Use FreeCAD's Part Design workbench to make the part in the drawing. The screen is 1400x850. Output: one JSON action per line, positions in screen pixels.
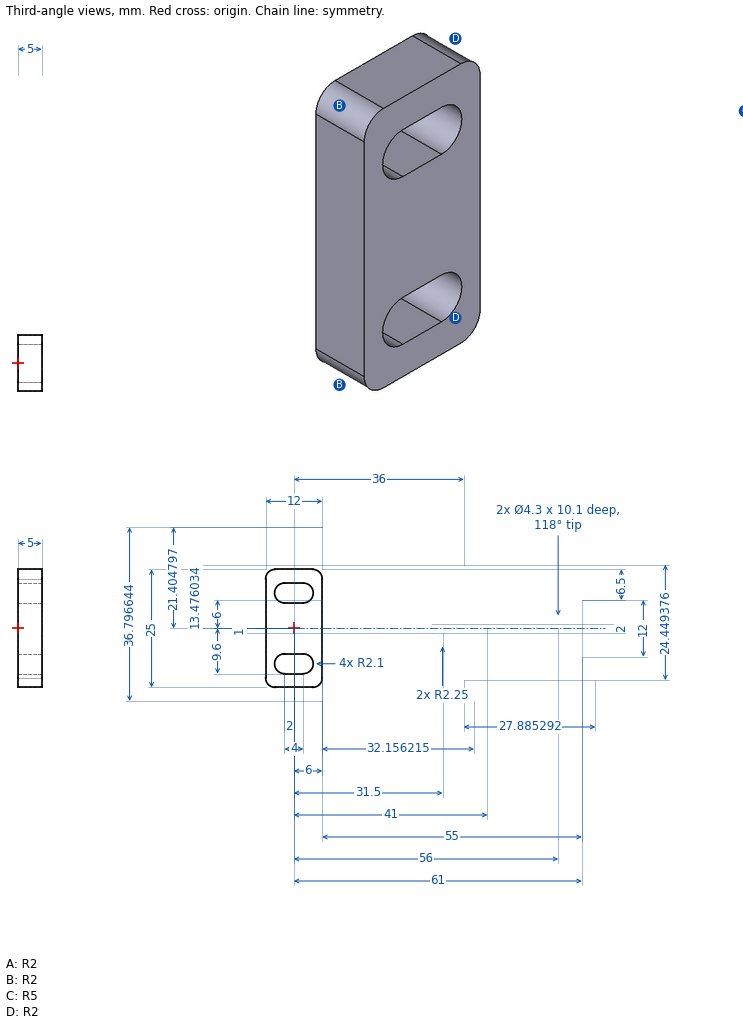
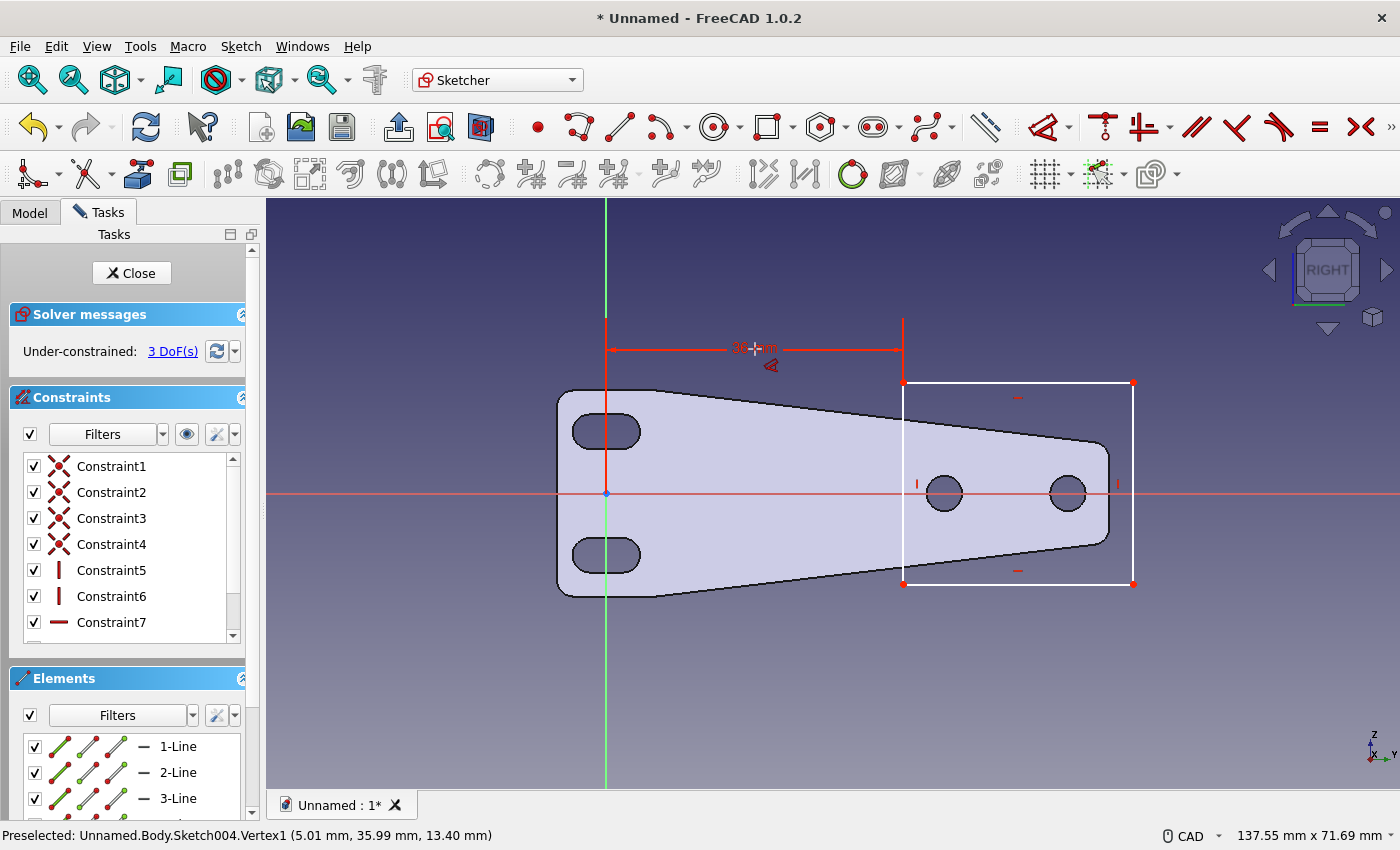
{"action": "left_click", "coordinate": [903, 444]}
{"action": "left_click", "coordinate": [937, 438]}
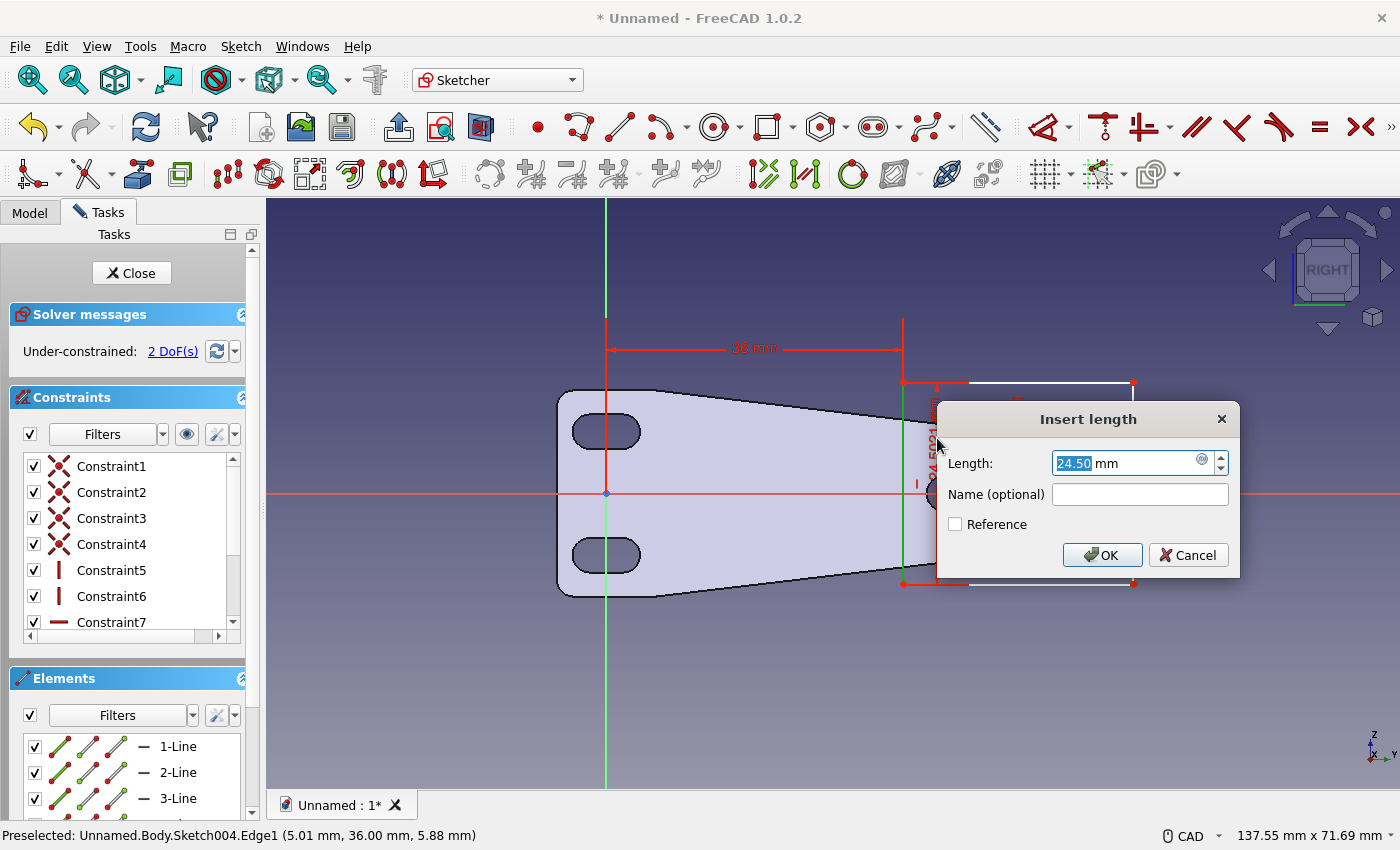
{"action": "type", "text": "24.449376"}
{"action": "key", "text": "Return"}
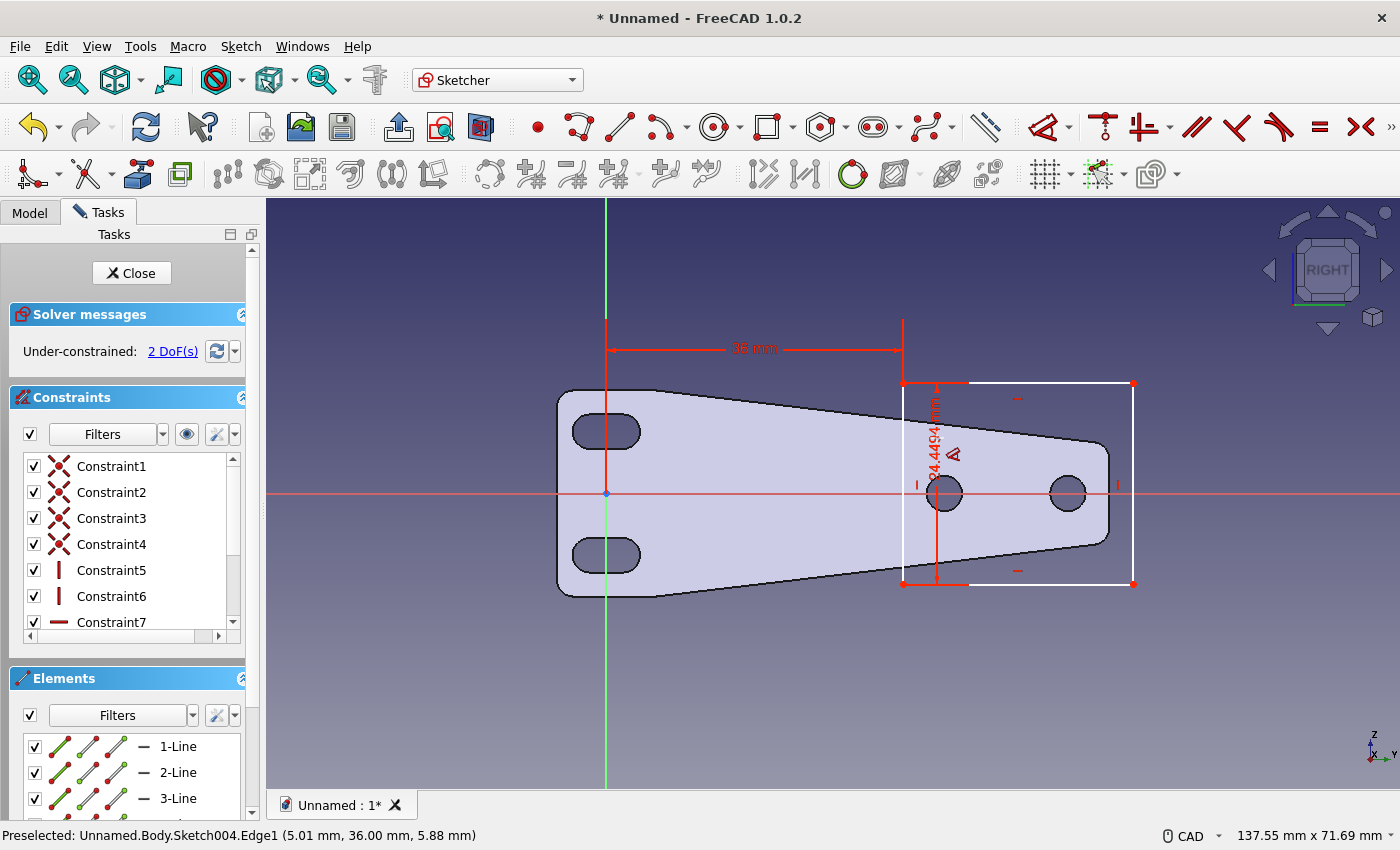
{"action": "left_click", "coordinate": [972, 585]}
{"action": "left_click", "coordinate": [1018, 619]}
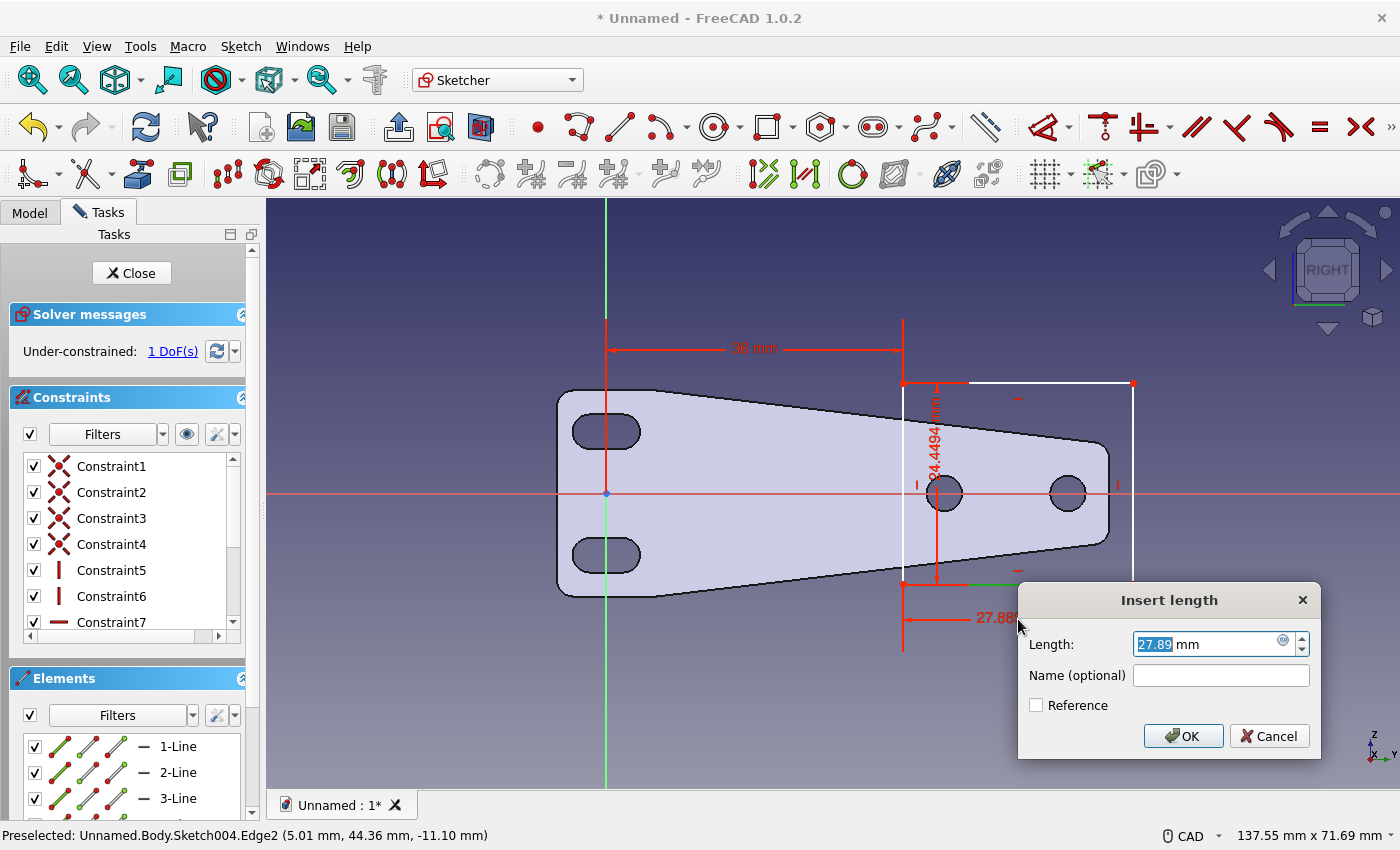
{"action": "type", "text": "27.885292"}
{"action": "key", "text": "Return"}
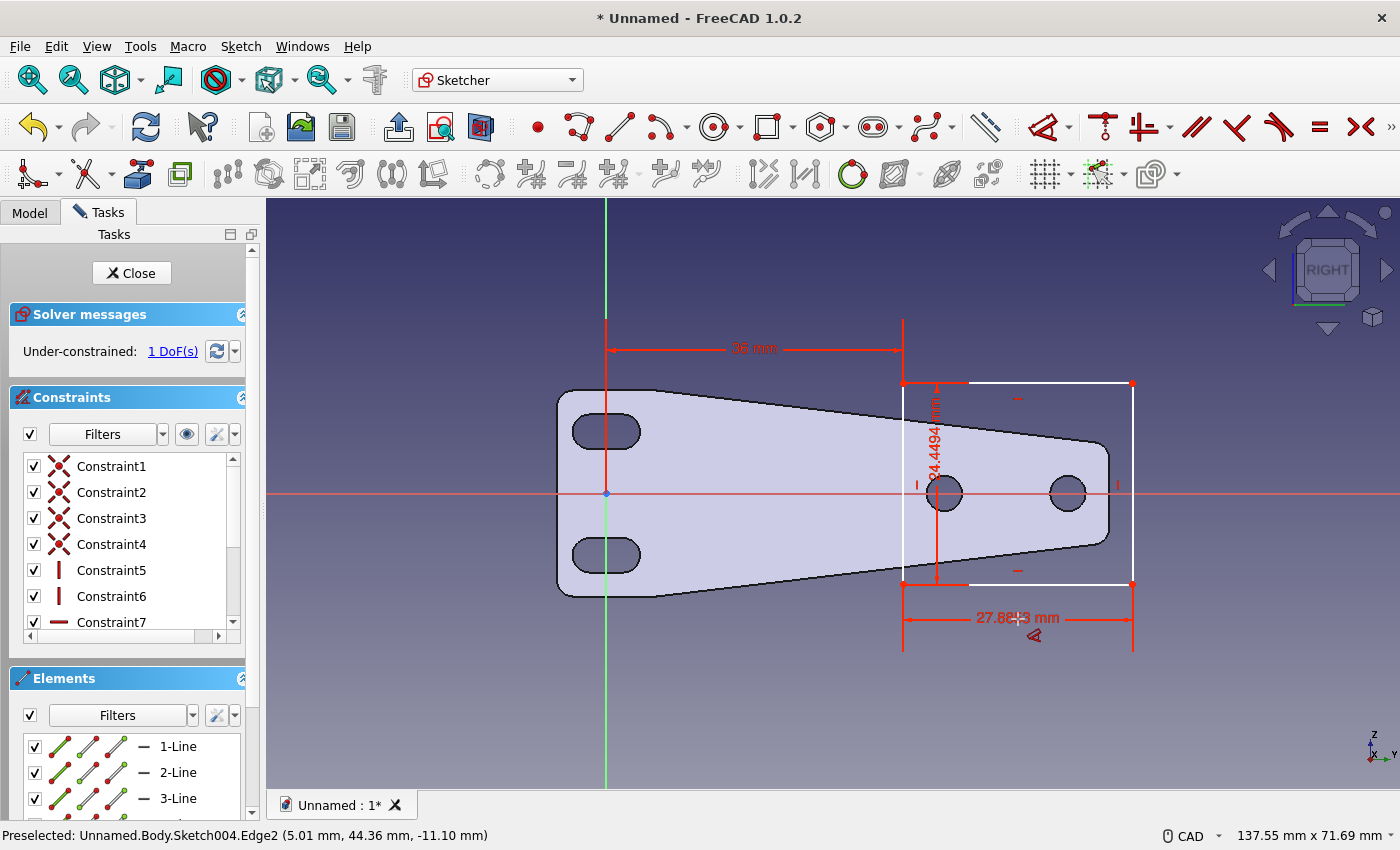
{"action": "left_click", "coordinate": [903, 383]}
{"action": "left_click", "coordinate": [572, 438]}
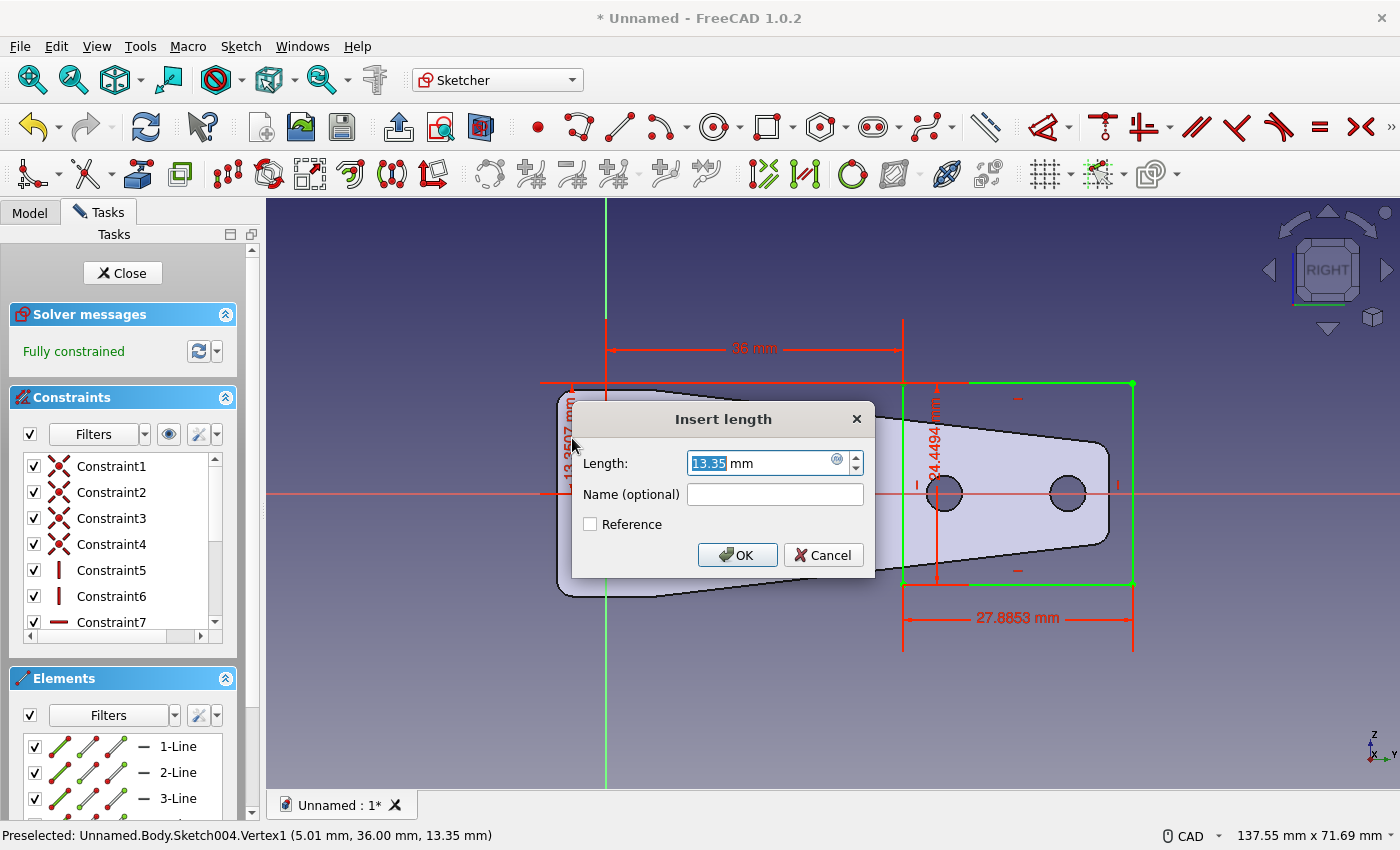
{"action": "type", "text": "13.476034"}
{"action": "key", "text": "Return"}
{"action": "key", "text": "Escape"}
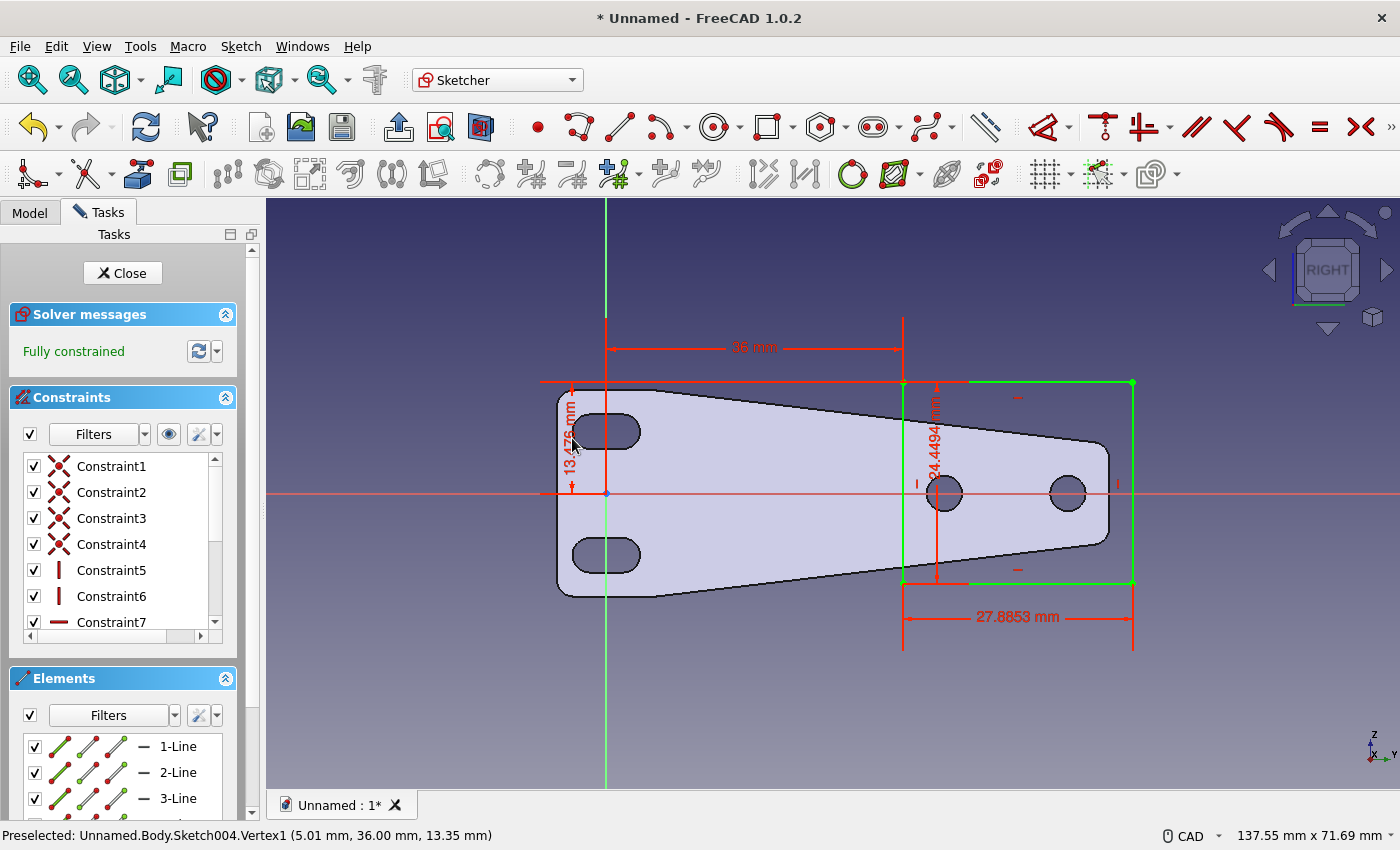
{"action": "left_click", "coordinate": [123, 273]}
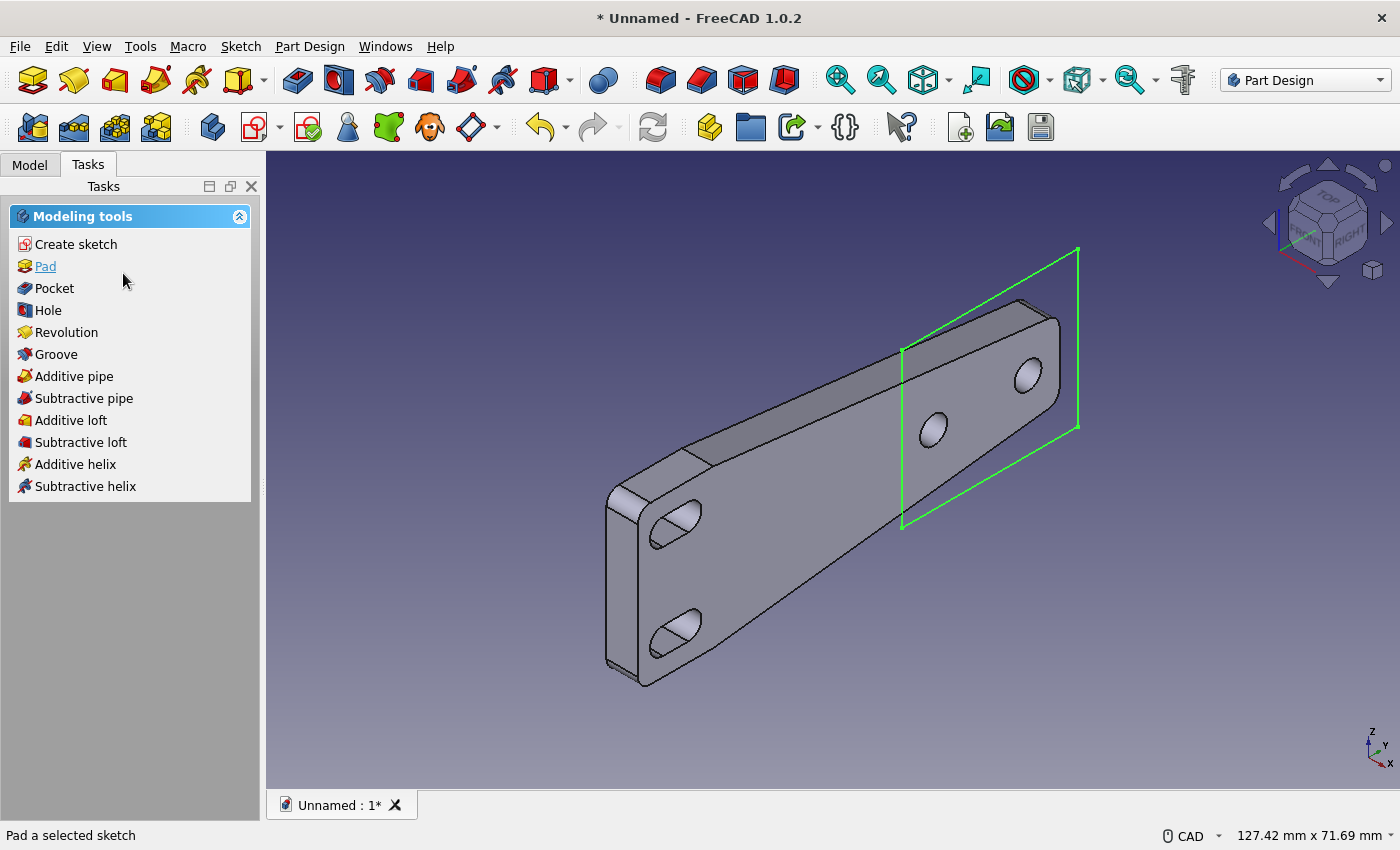
{"action": "left_click", "coordinate": [298, 80]}